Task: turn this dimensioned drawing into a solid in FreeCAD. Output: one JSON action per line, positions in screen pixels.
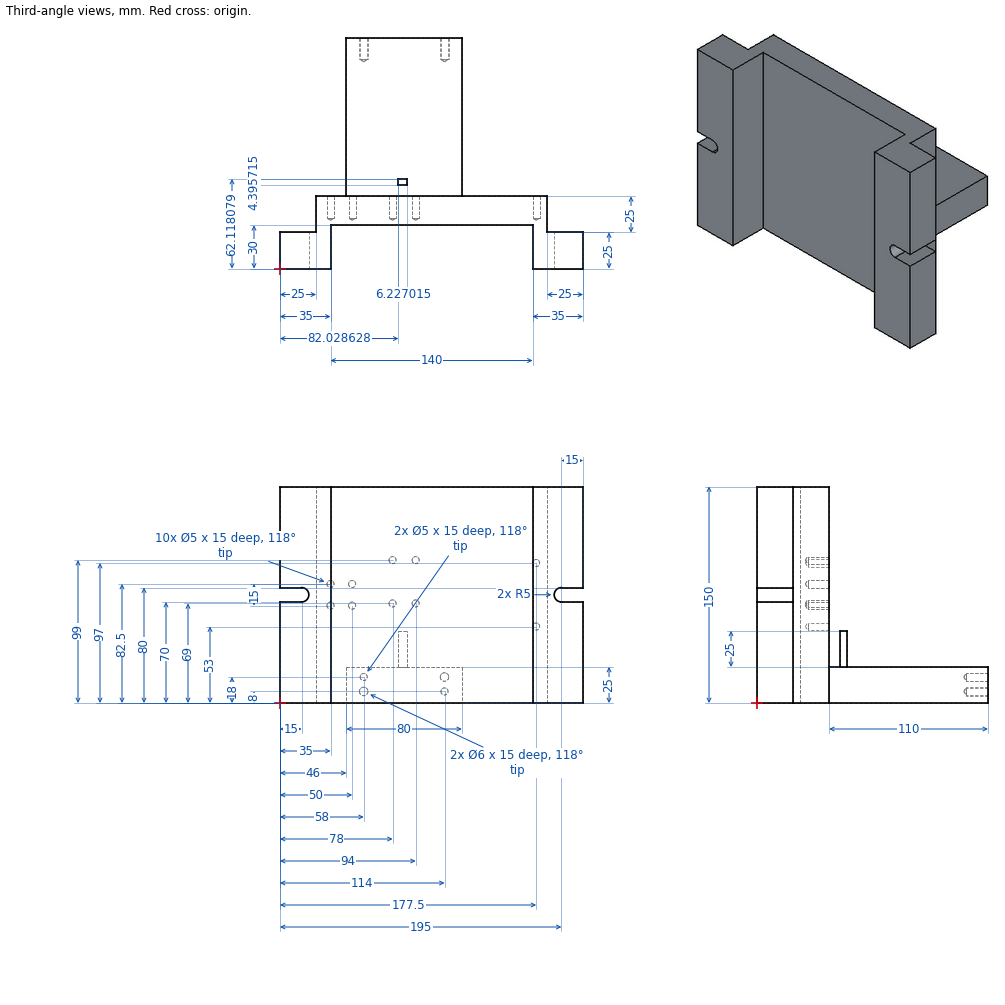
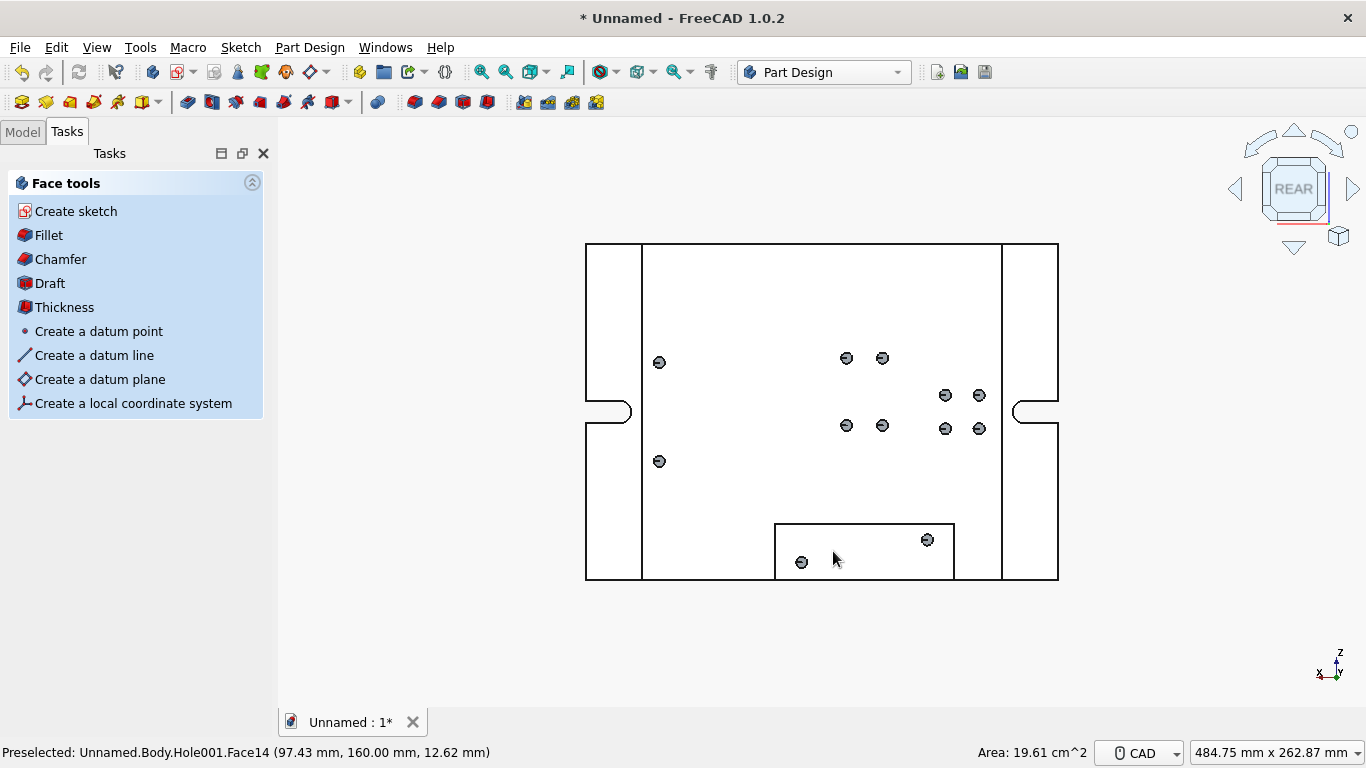
{"action": "left_click", "coordinate": [178, 72]}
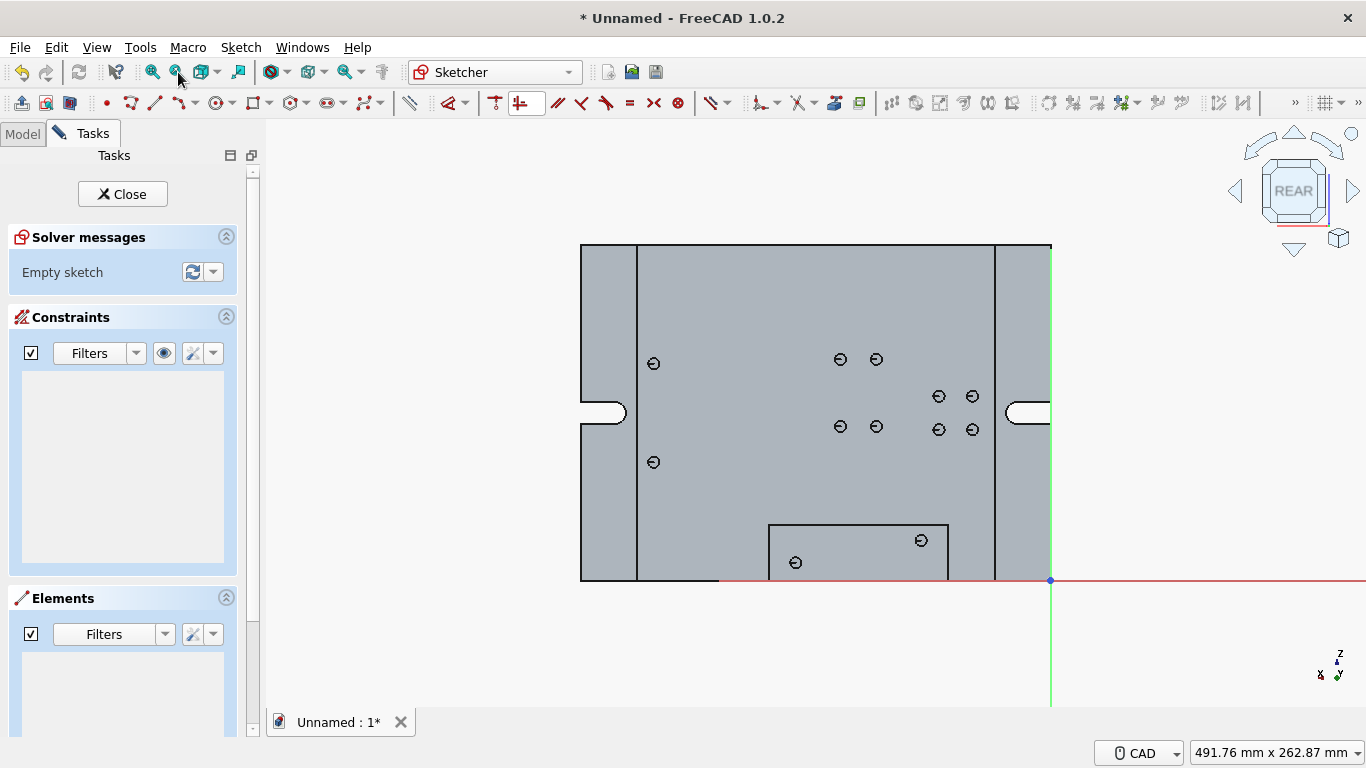
{"action": "scroll", "coordinate": [1061, 675], "scroll_direction": "up", "scroll_amount": 4}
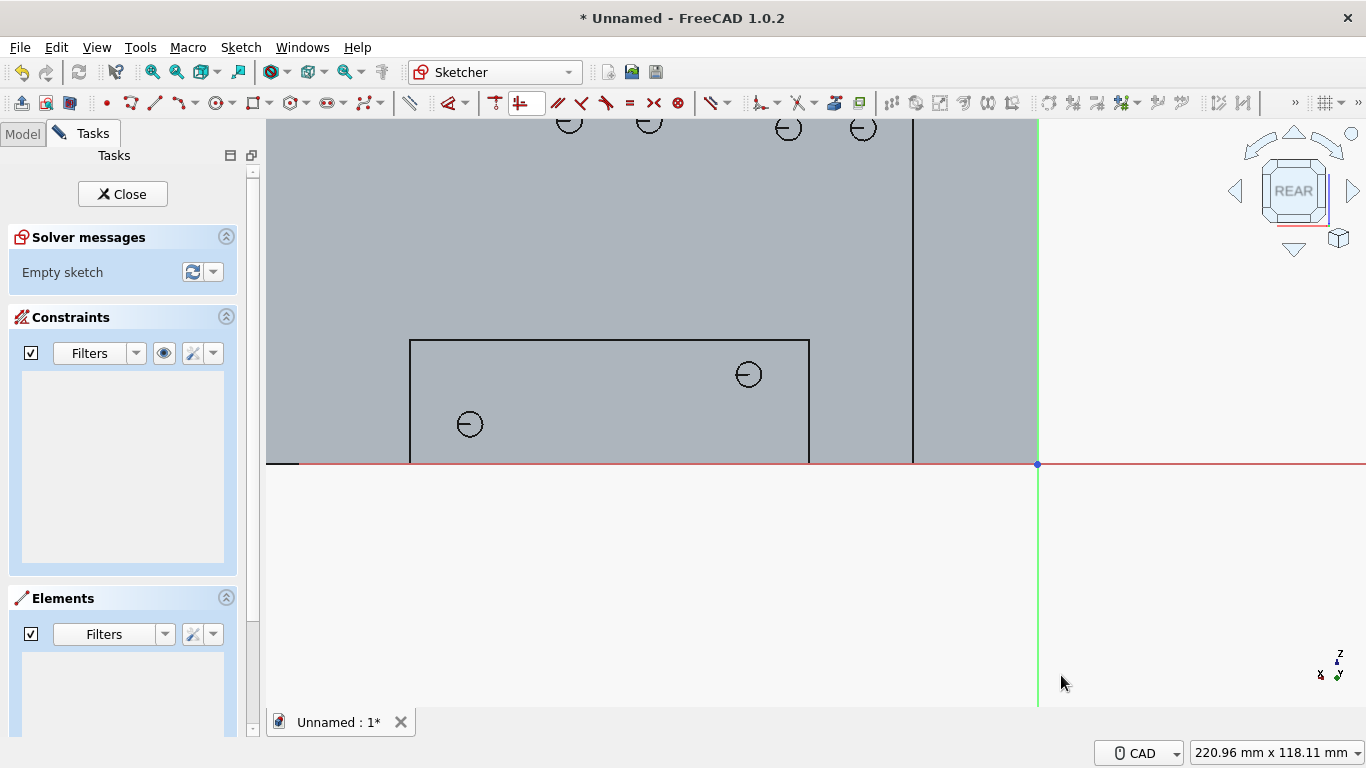
{"action": "left_click", "coordinate": [216, 104]}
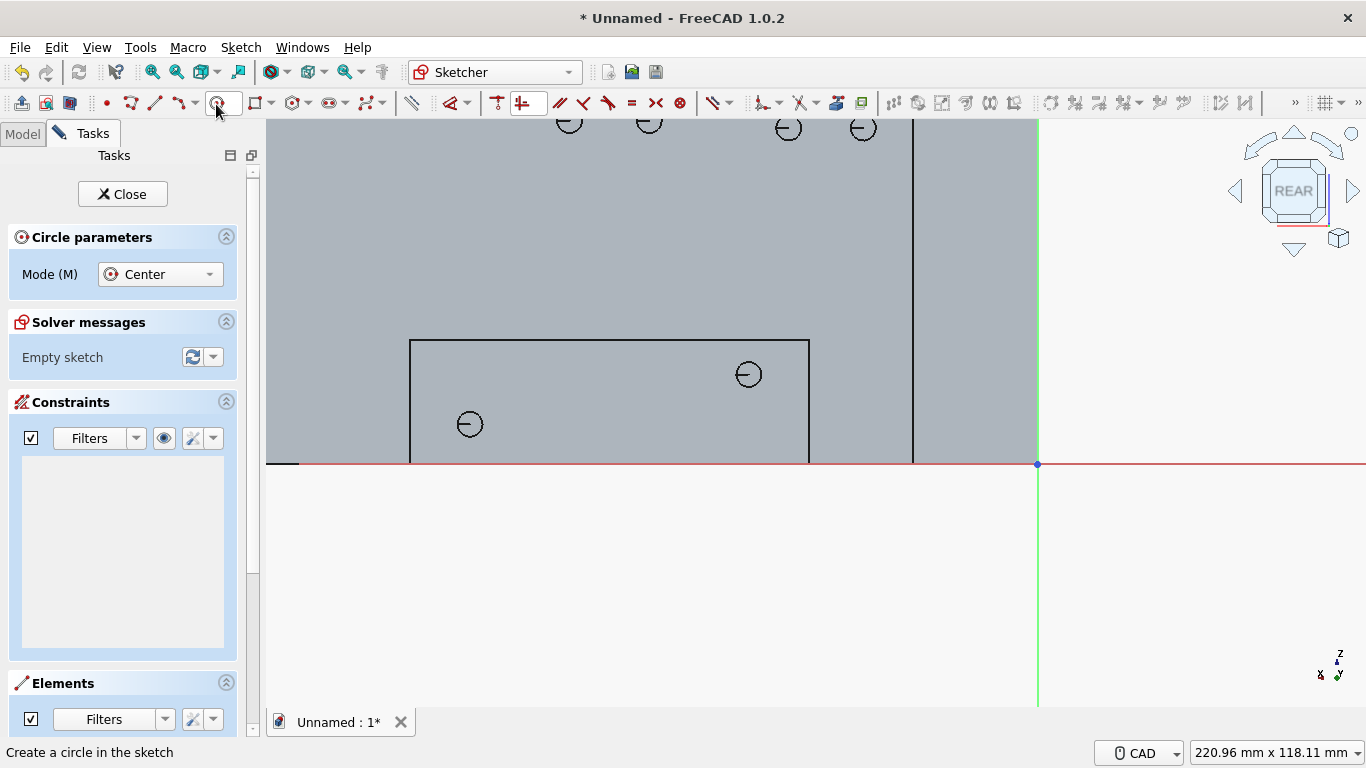
{"action": "scroll", "coordinate": [749, 424], "scroll_direction": "up", "scroll_amount": 3}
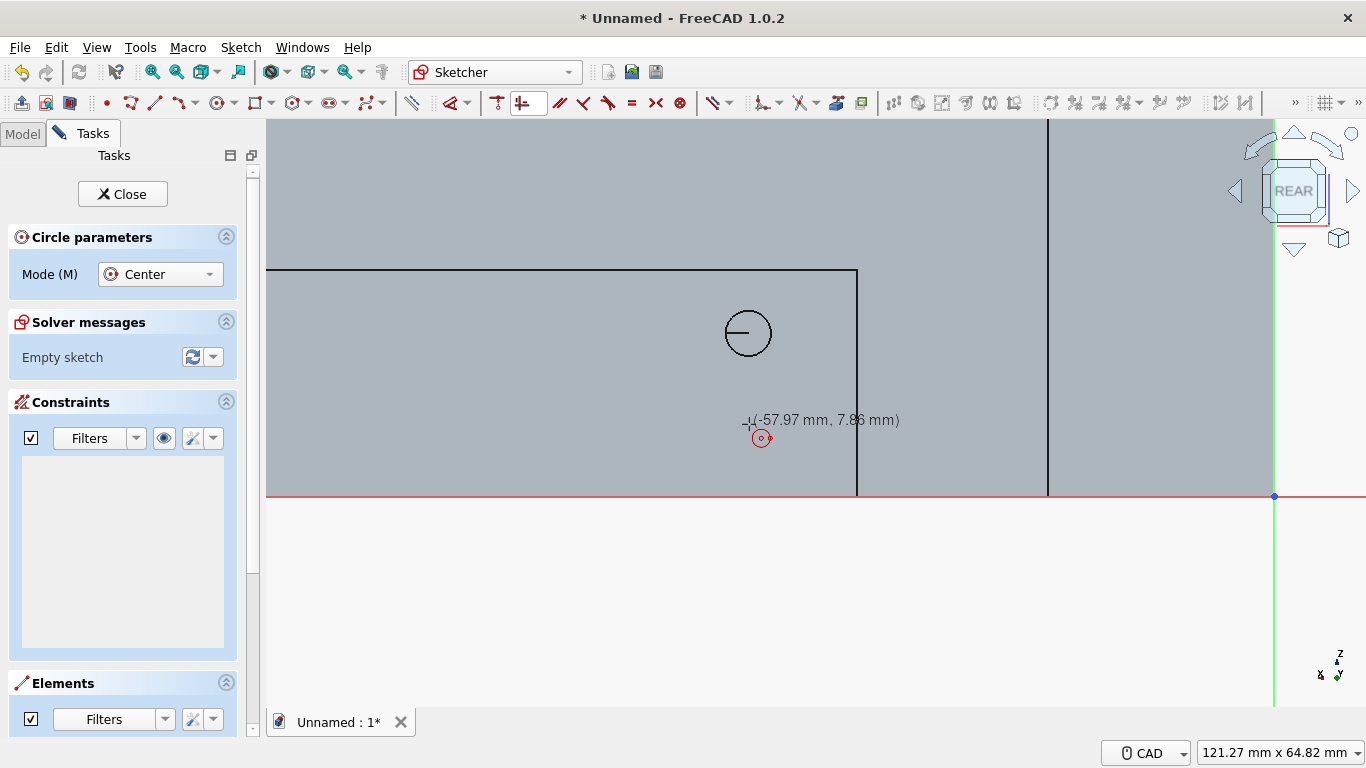
{"action": "left_click", "coordinate": [748, 424]}
{"action": "mouse_move", "coordinate": [768, 405]}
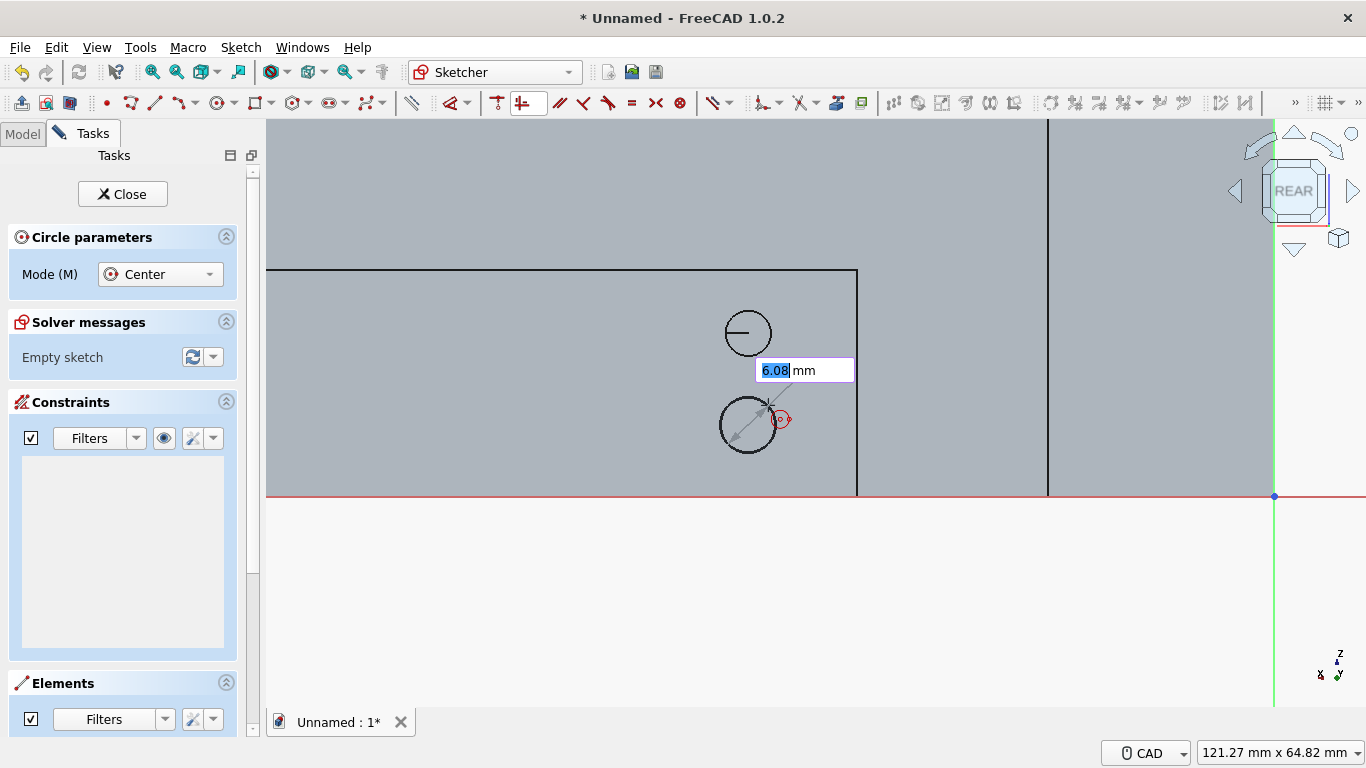
{"action": "type", "text": "6"}
{"action": "key", "text": "Return"}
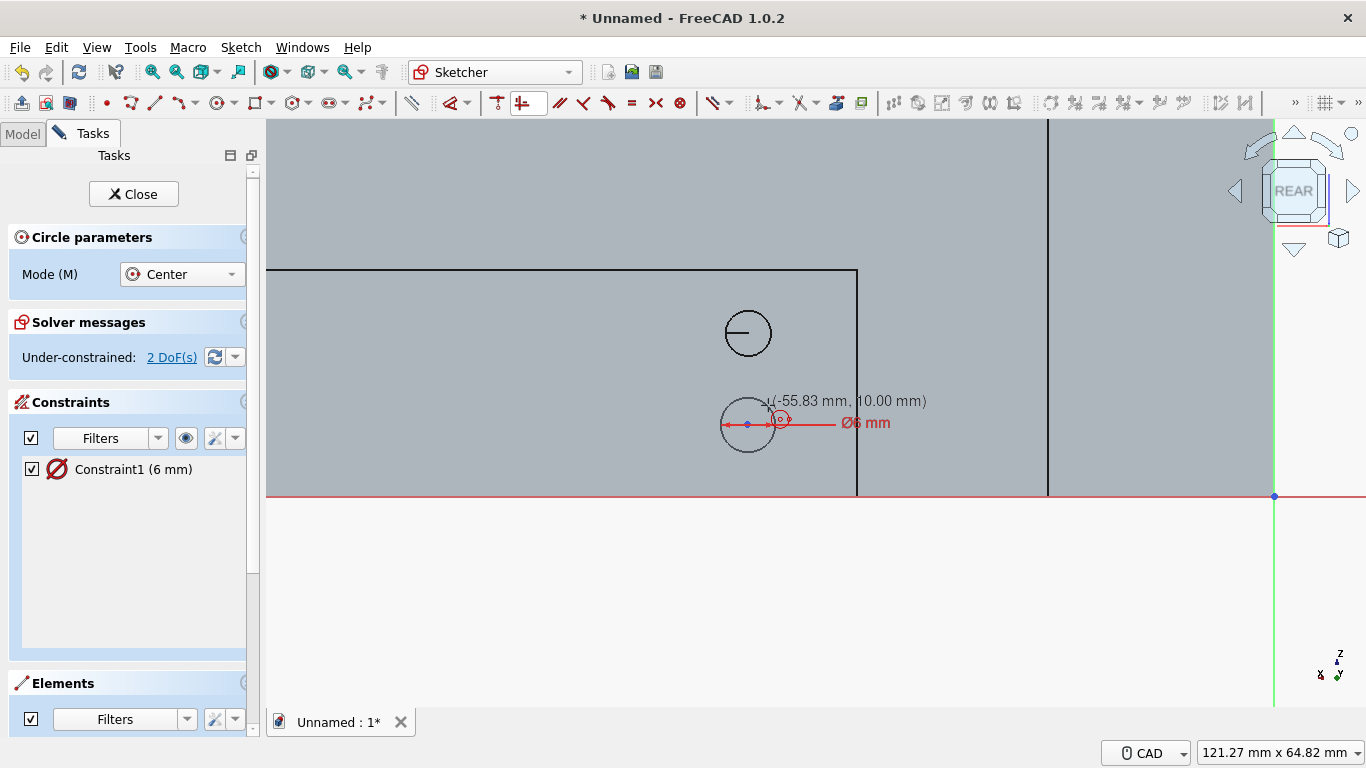
{"action": "scroll", "coordinate": [752, 427], "scroll_direction": "down", "scroll_amount": 3}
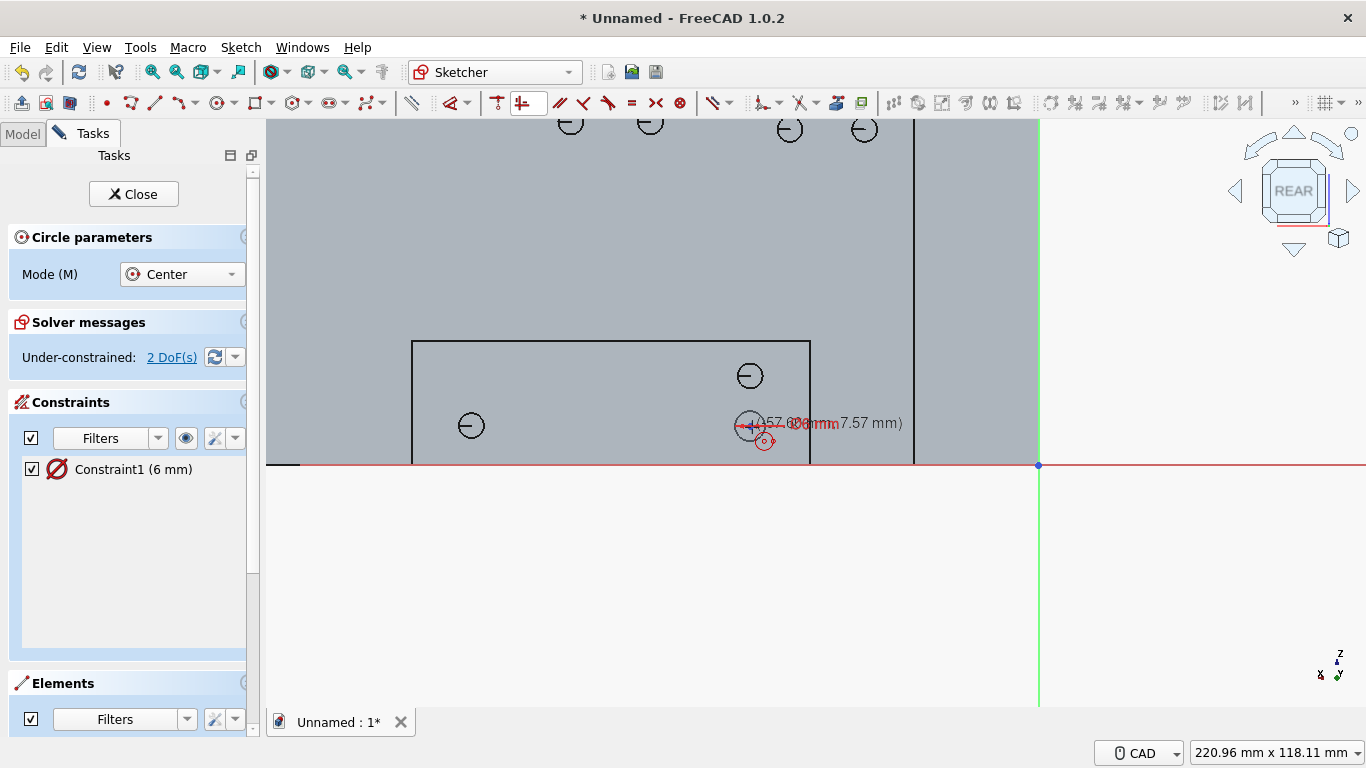
{"action": "scroll", "coordinate": [471, 376], "scroll_direction": "up", "scroll_amount": 3}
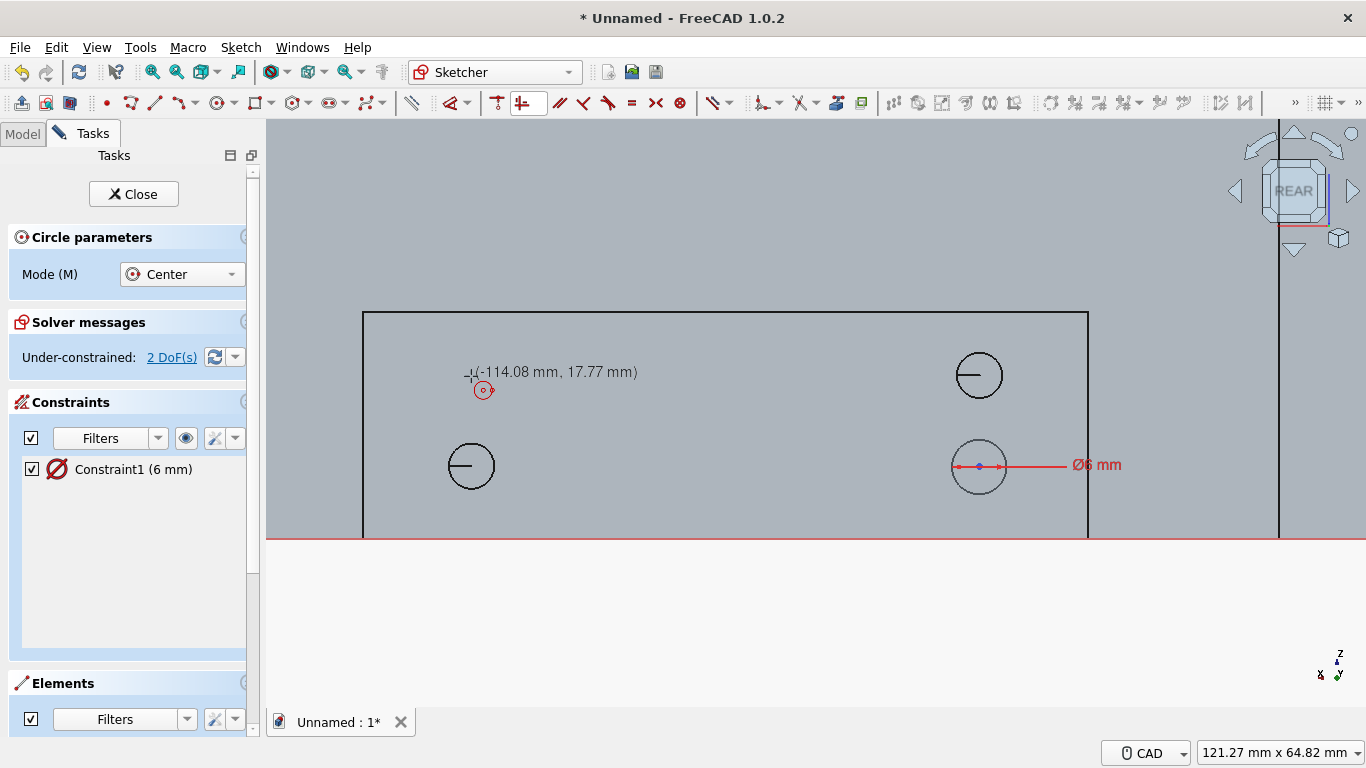
{"action": "left_click", "coordinate": [472, 375]}
{"action": "mouse_move", "coordinate": [491, 356]}